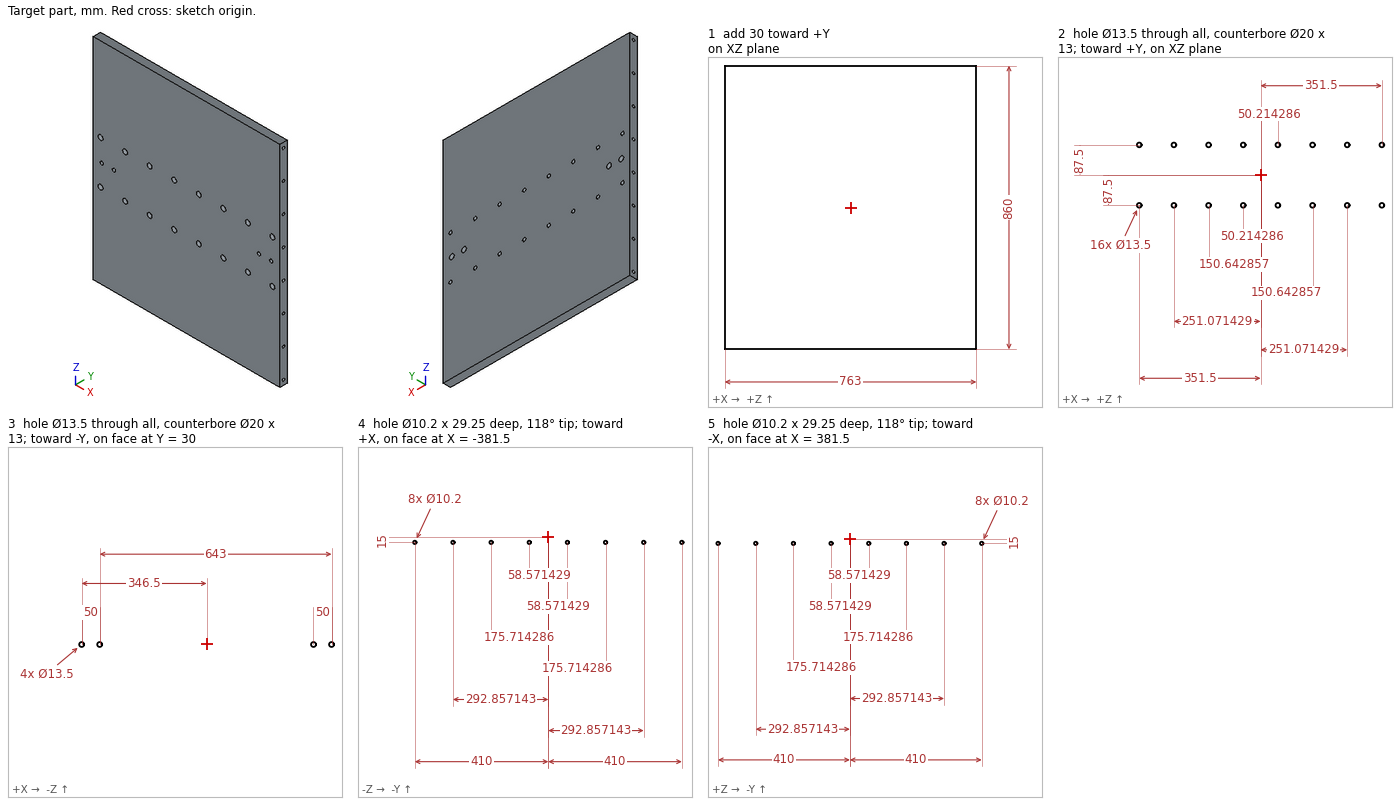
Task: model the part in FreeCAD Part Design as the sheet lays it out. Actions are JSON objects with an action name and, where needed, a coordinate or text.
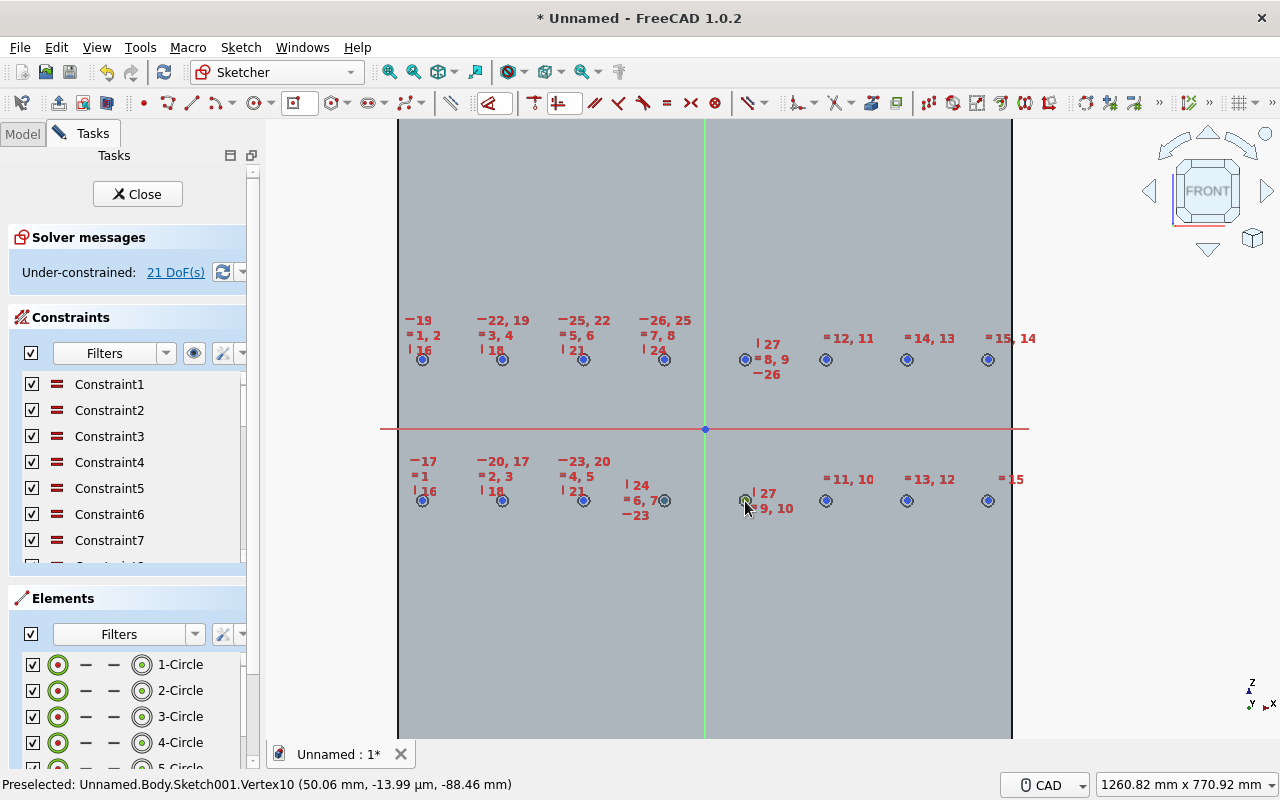
{"action": "key", "text": "h"}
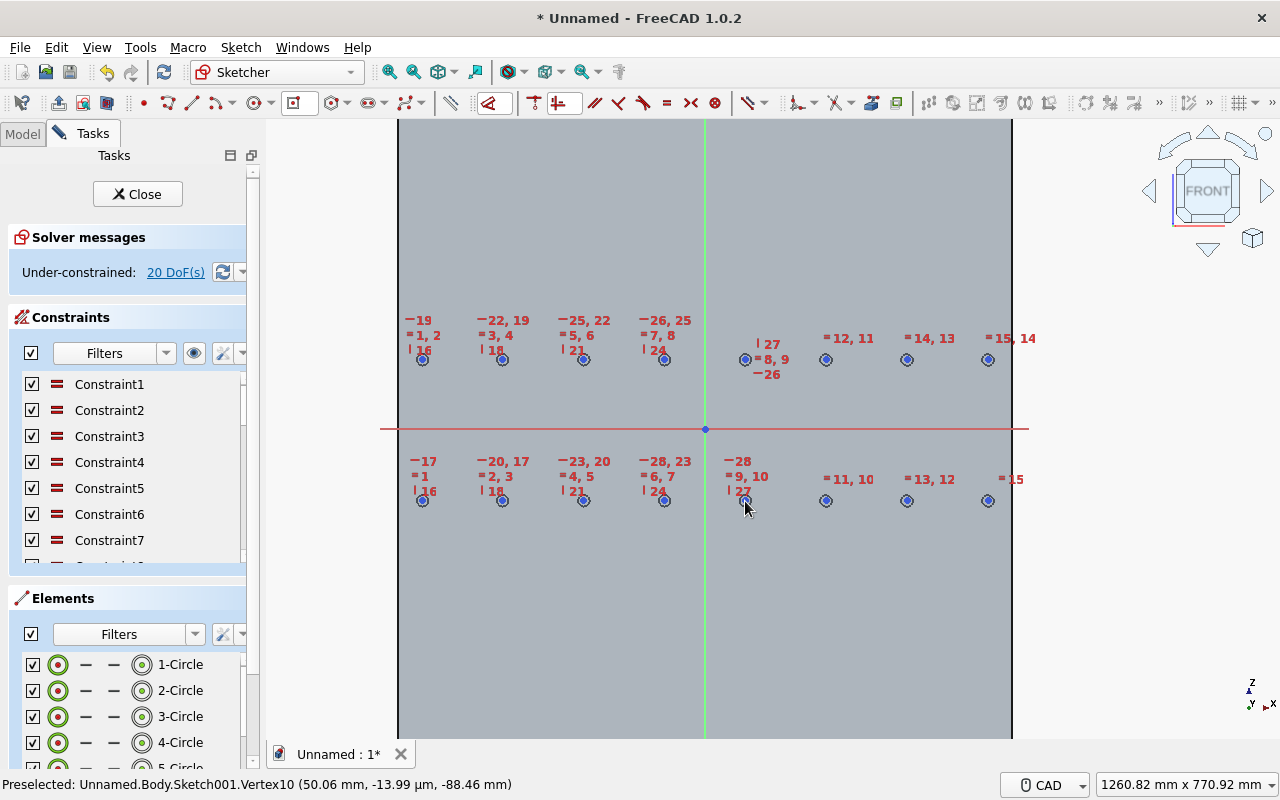
{"action": "left_click", "coordinate": [745, 501]}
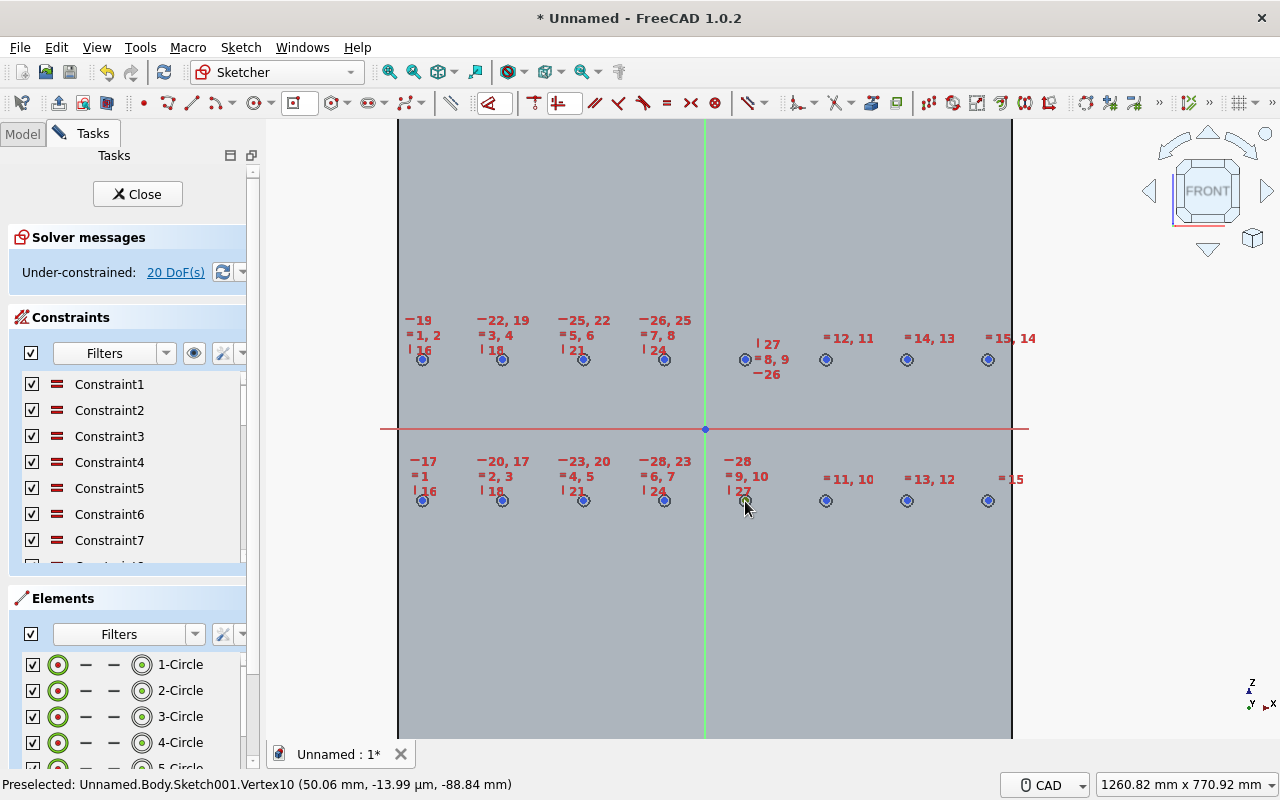
{"action": "left_click", "coordinate": [826, 501]}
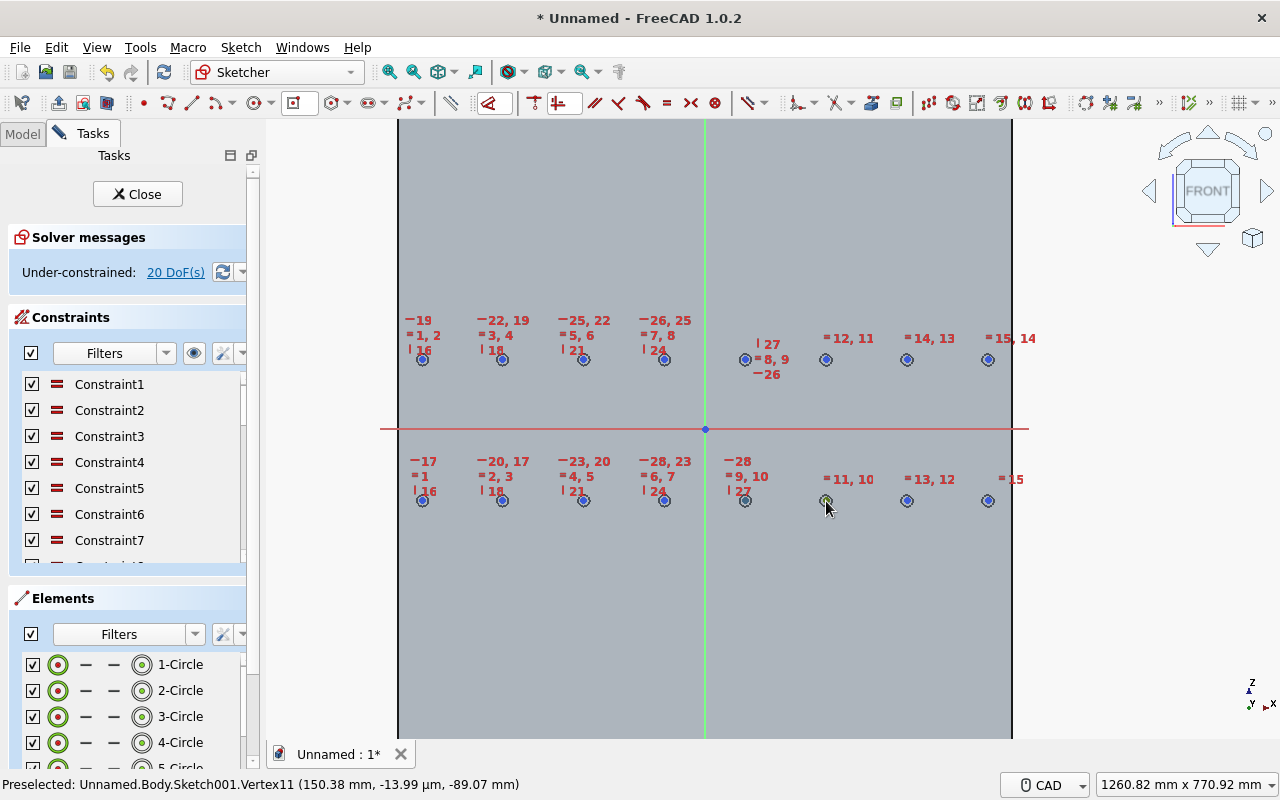
{"action": "left_click", "coordinate": [576, 104]}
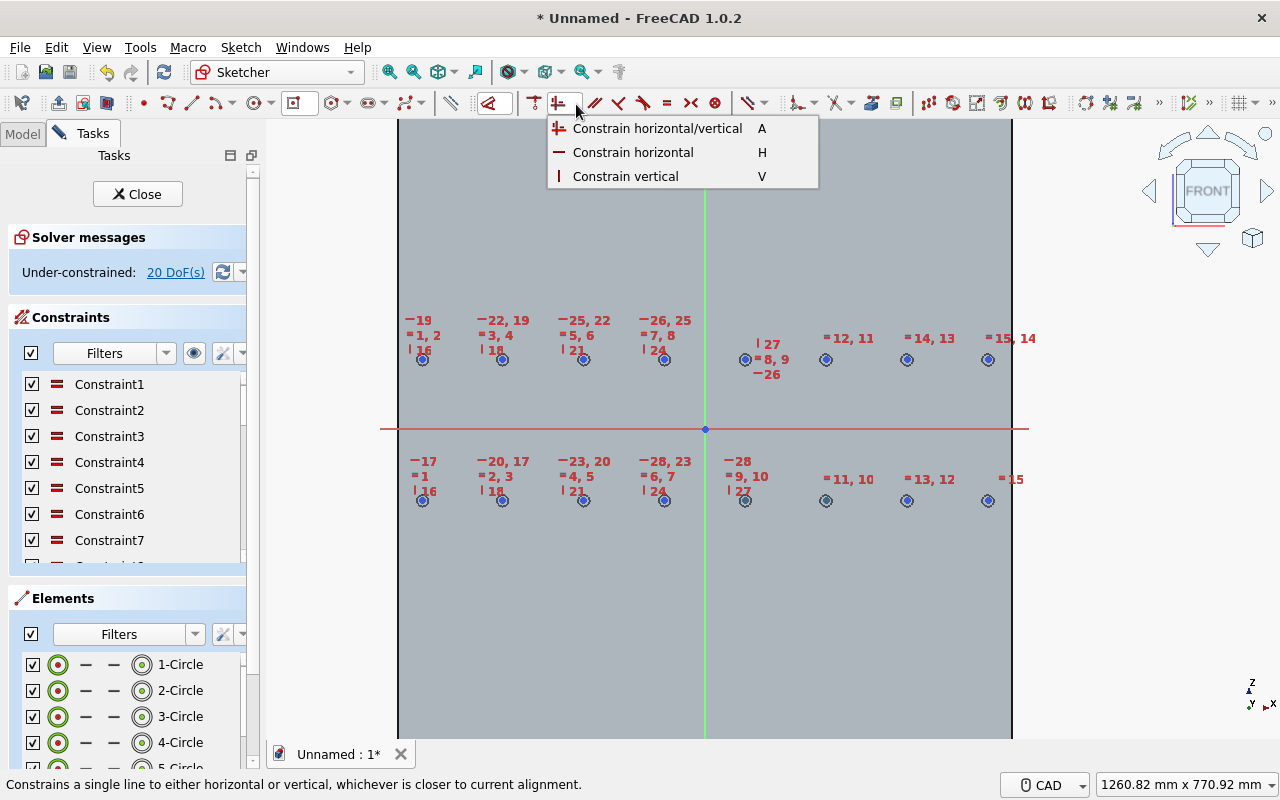
{"action": "left_click", "coordinate": [683, 152]}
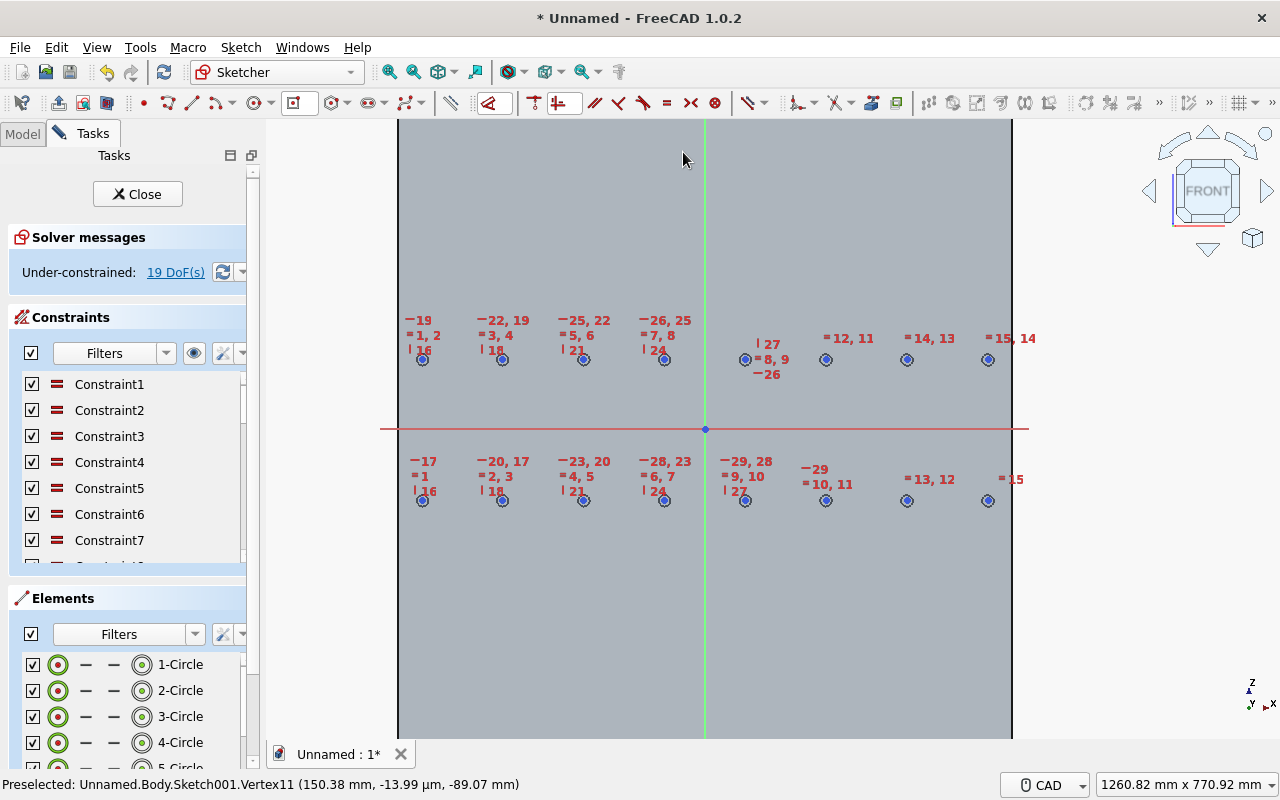
{"action": "left_click", "coordinate": [826, 501]}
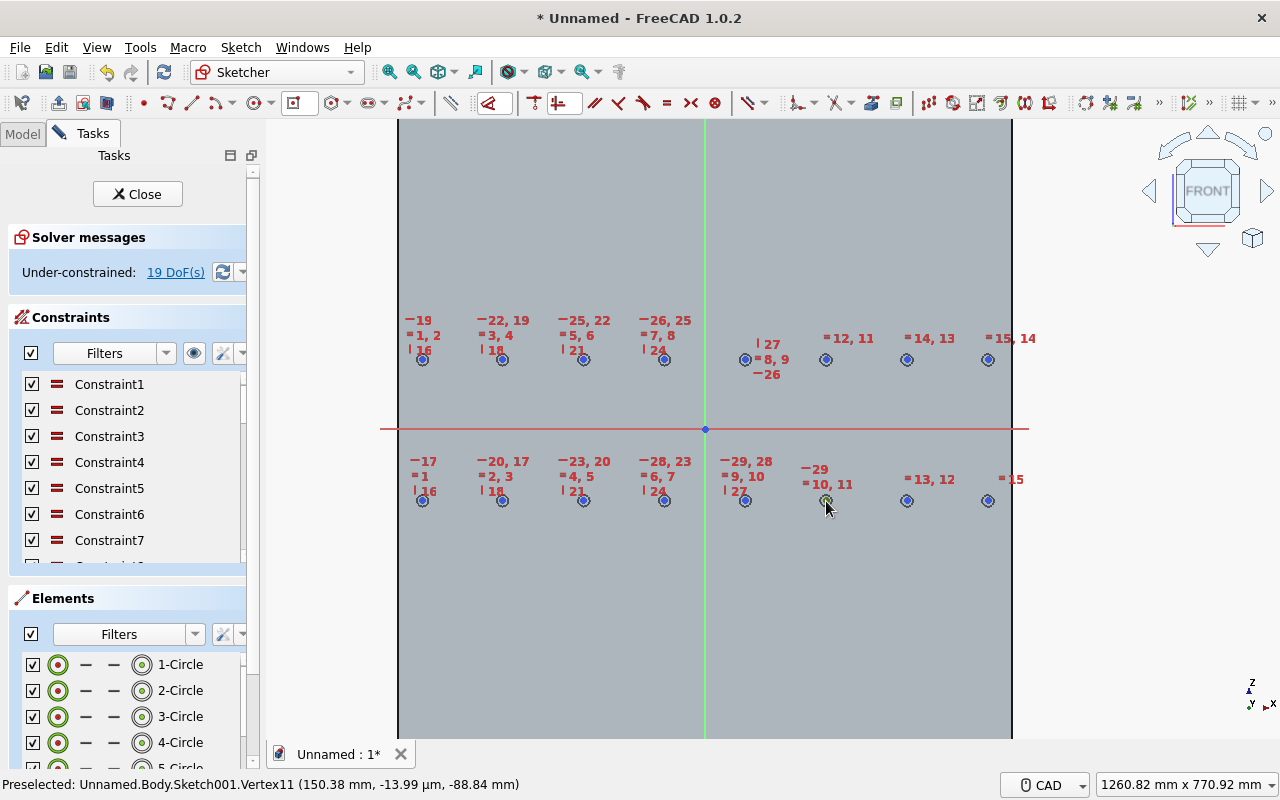
{"action": "left_click", "coordinate": [826, 360]}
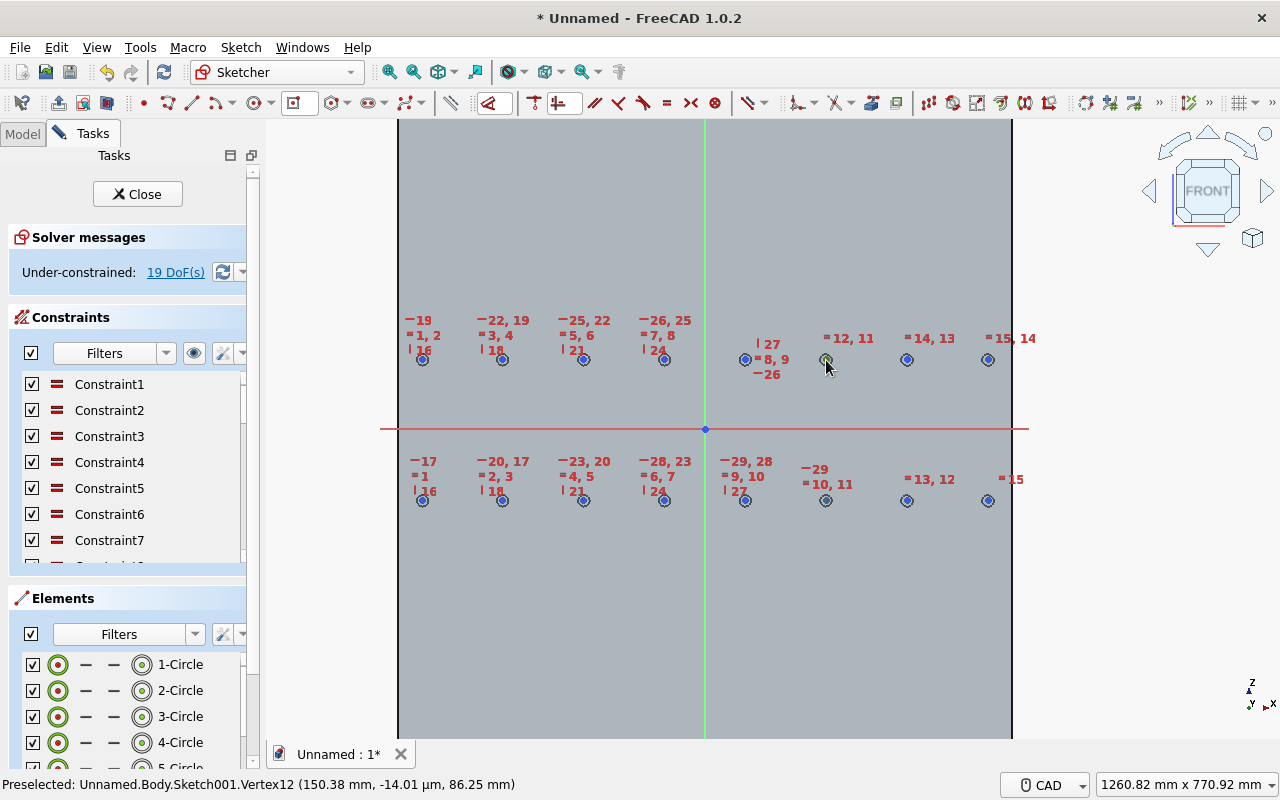
{"action": "key", "text": "v"}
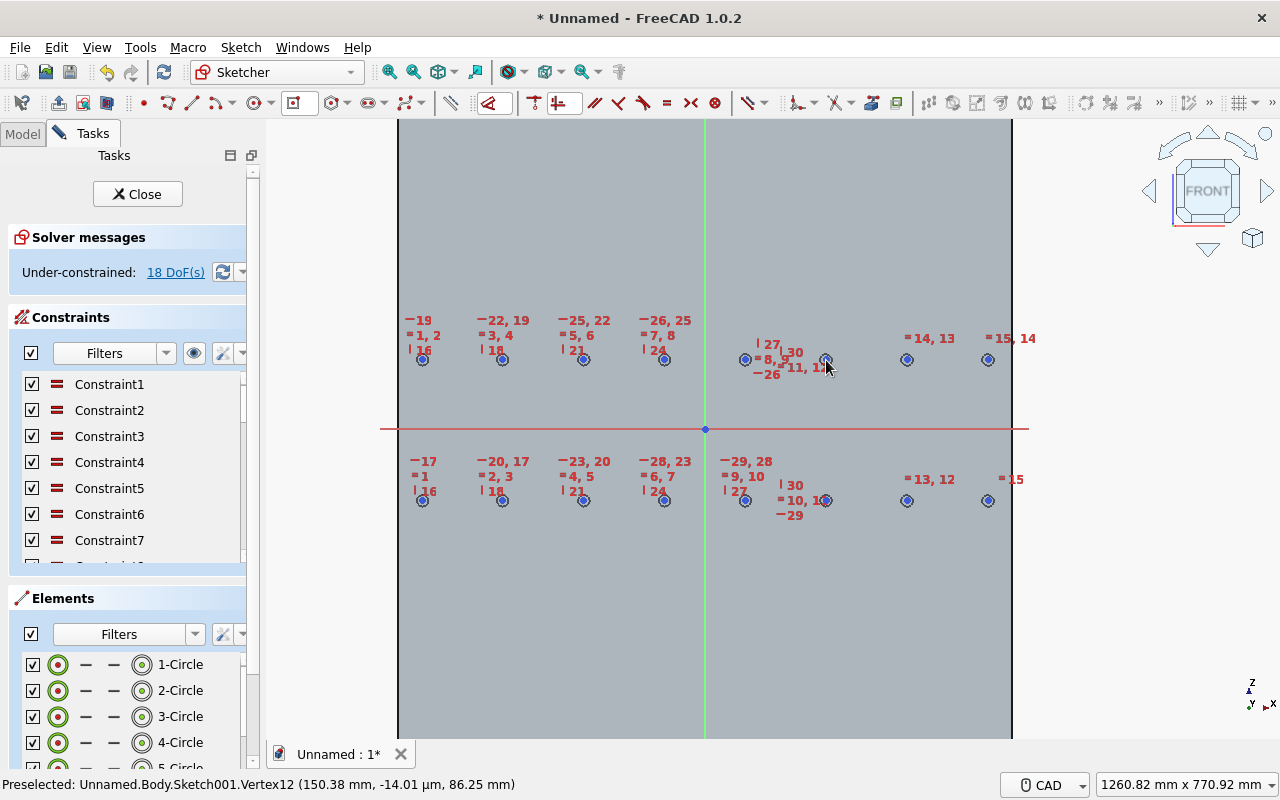
{"action": "left_click", "coordinate": [745, 360]}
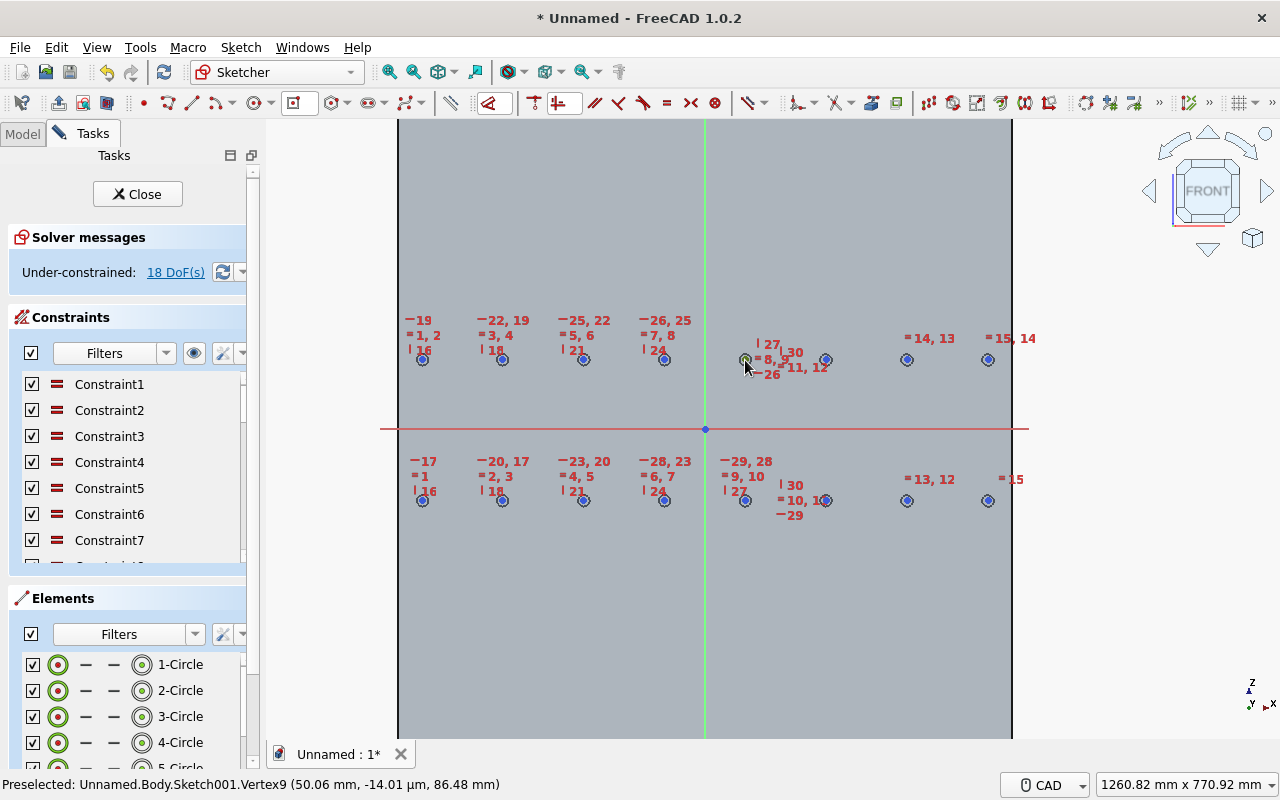
{"action": "left_click", "coordinate": [828, 362]}